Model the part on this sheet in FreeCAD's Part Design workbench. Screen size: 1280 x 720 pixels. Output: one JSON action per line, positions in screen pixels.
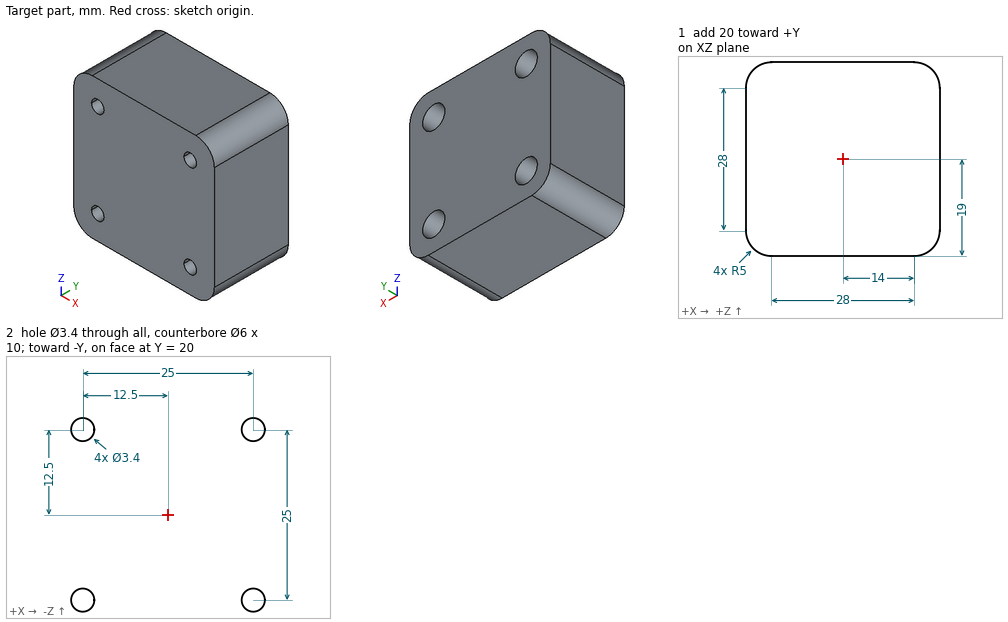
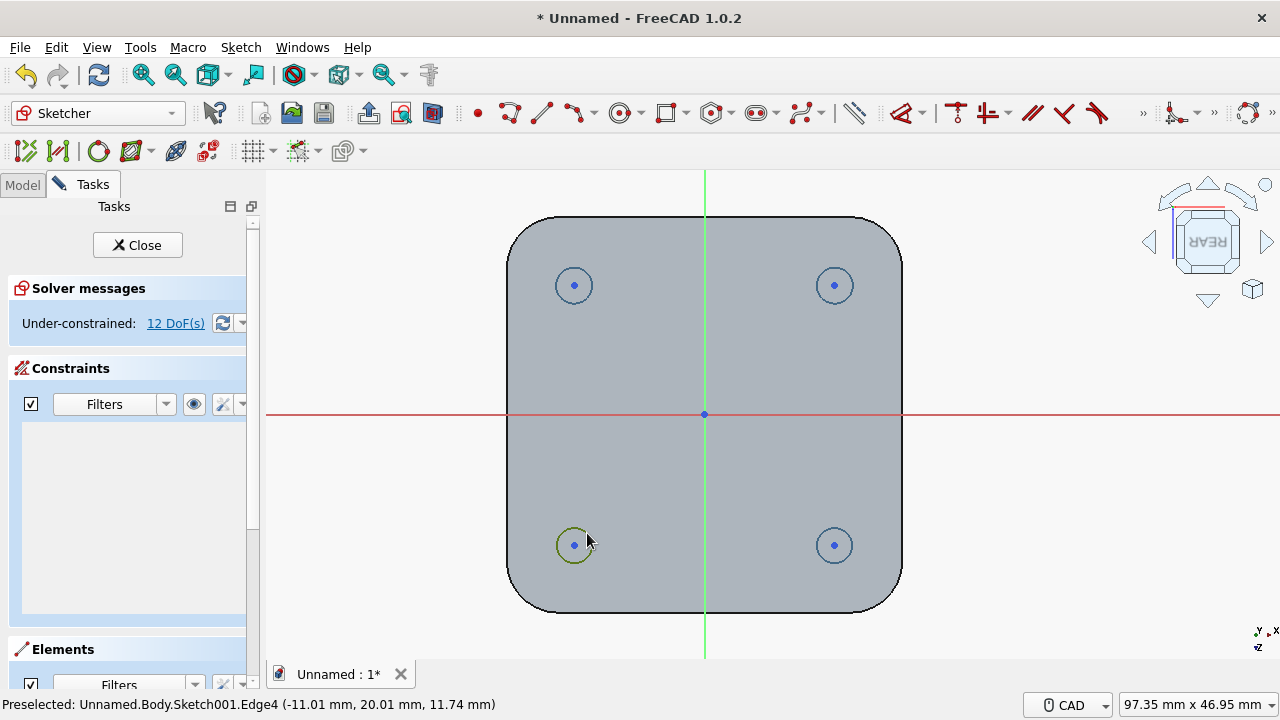
{"action": "key", "text": "e"}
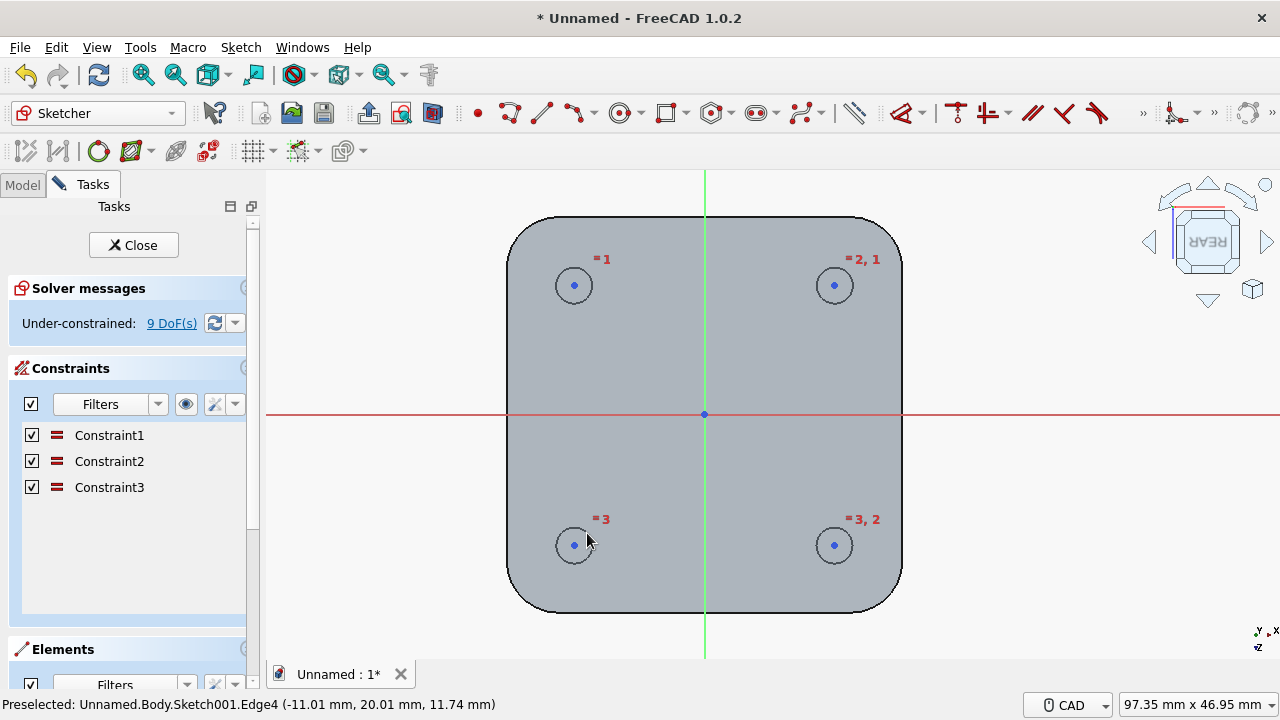
{"action": "left_click", "coordinate": [574, 286]}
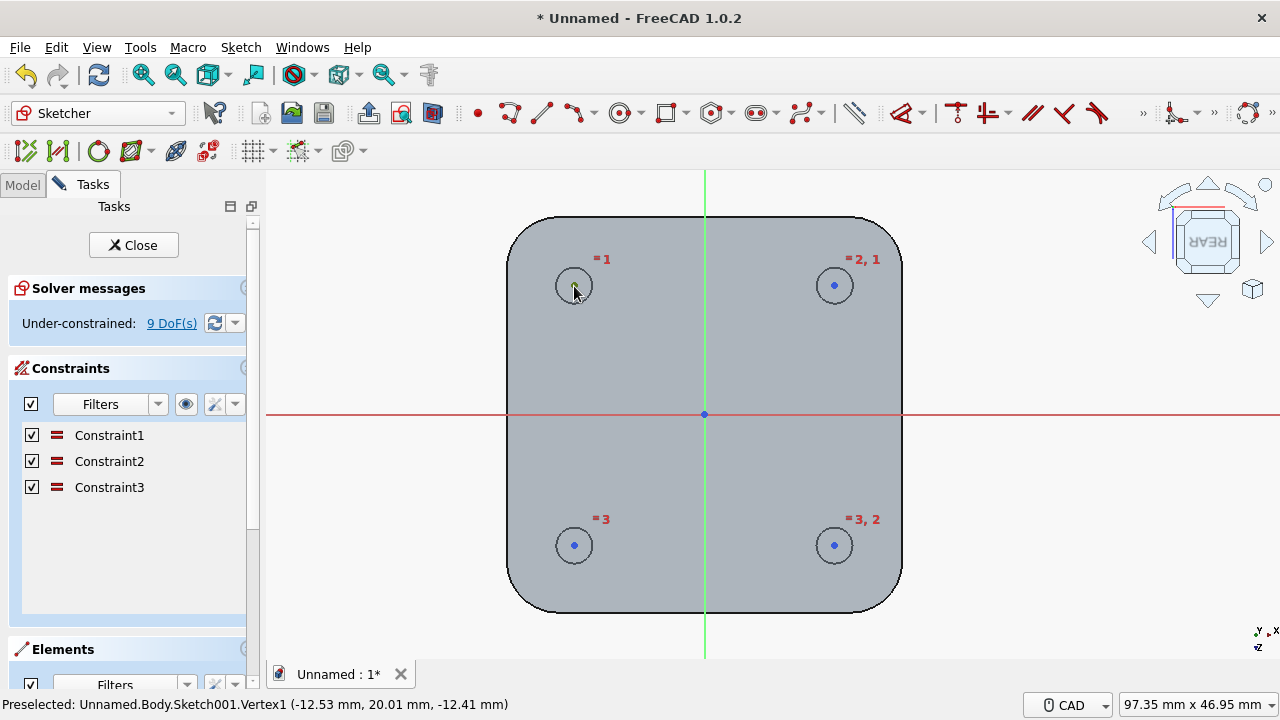
{"action": "left_click", "coordinate": [835, 286]}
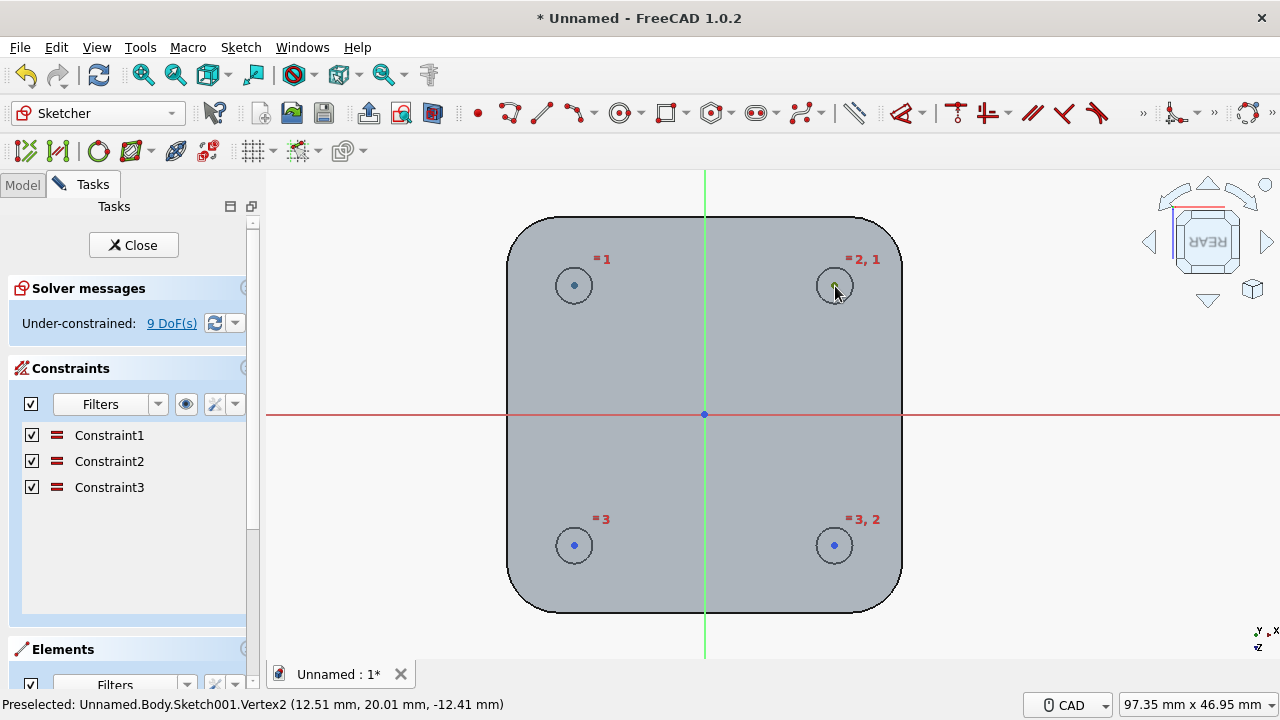
{"action": "left_click", "coordinate": [1010, 114]}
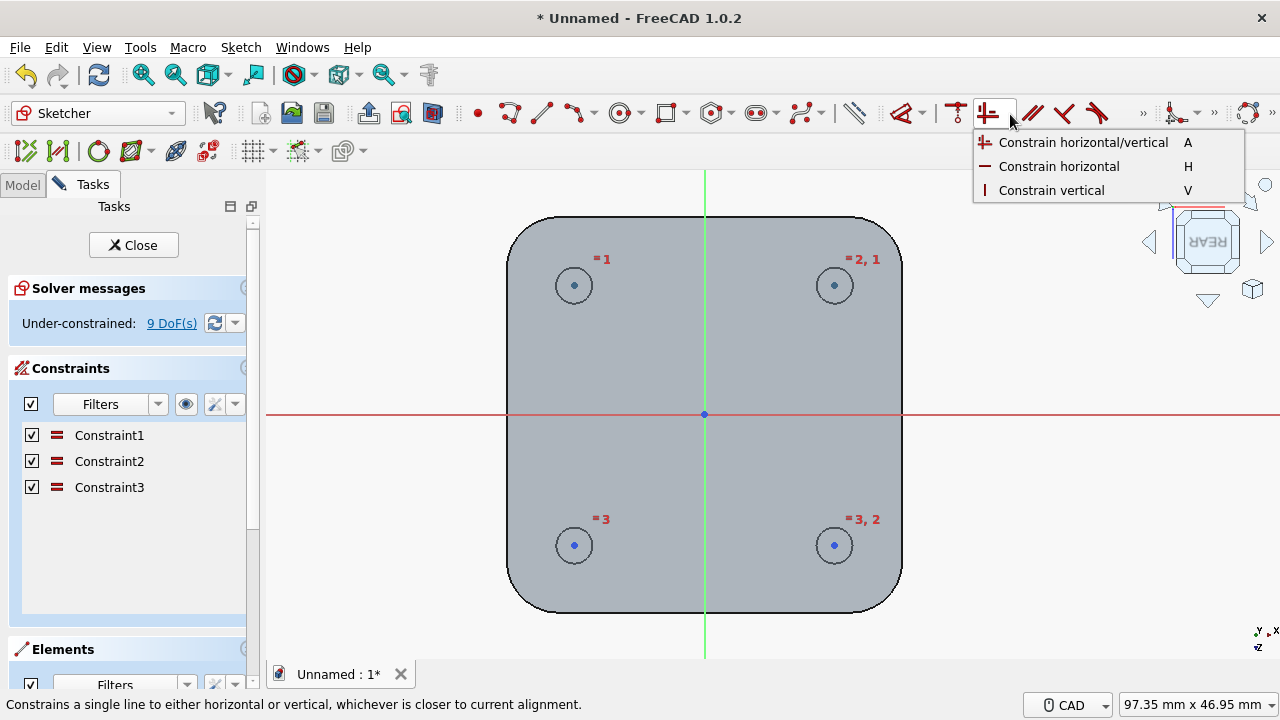
{"action": "left_click", "coordinate": [1109, 166]}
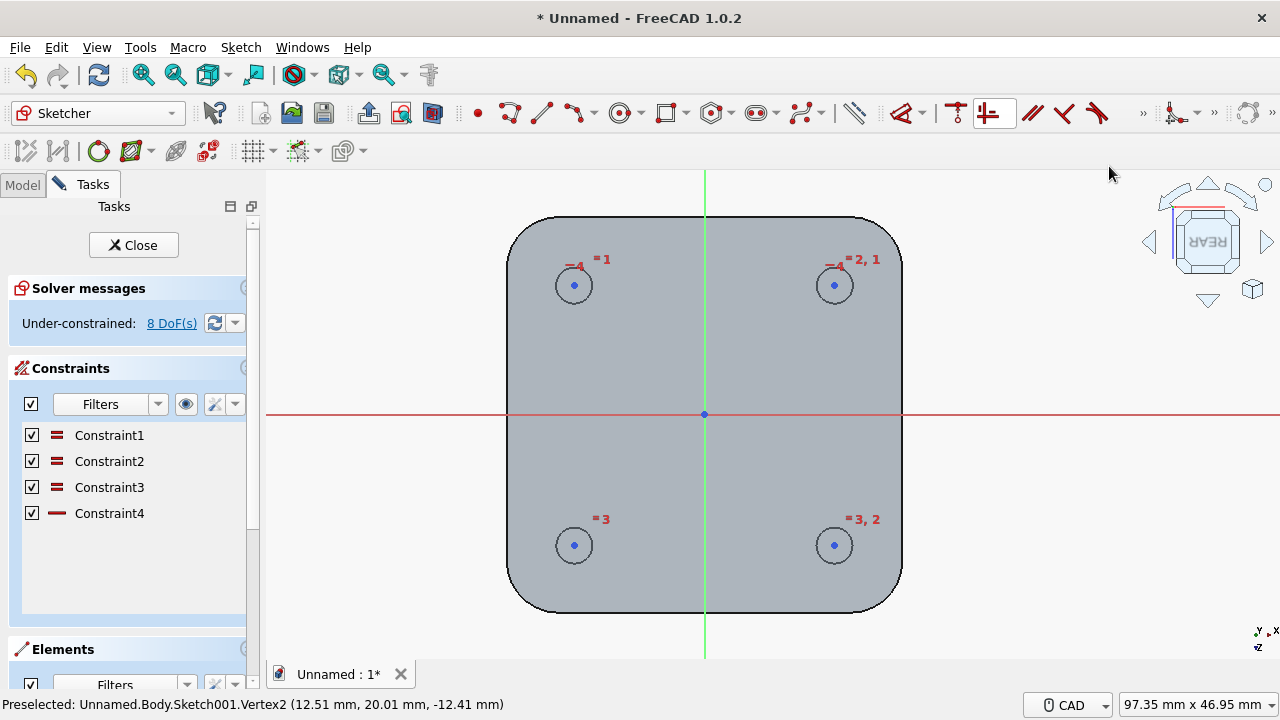
{"action": "left_click", "coordinate": [835, 286]}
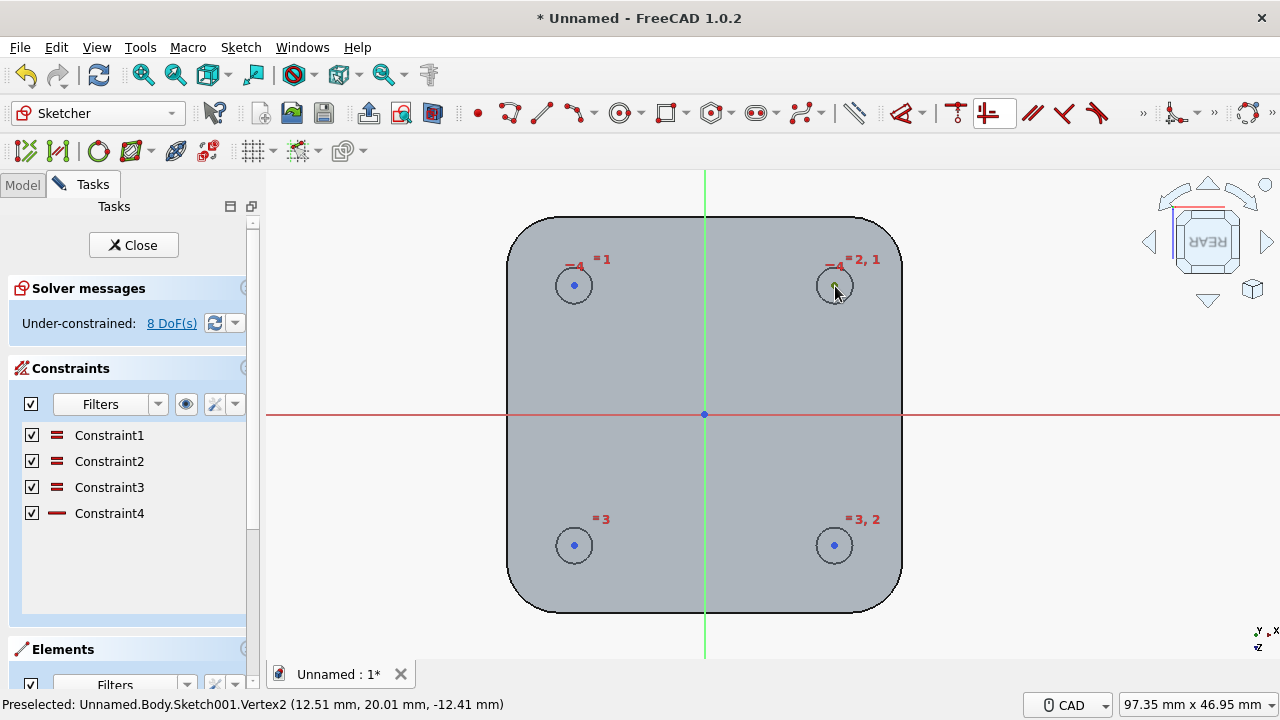
{"action": "left_click", "coordinate": [835, 546]}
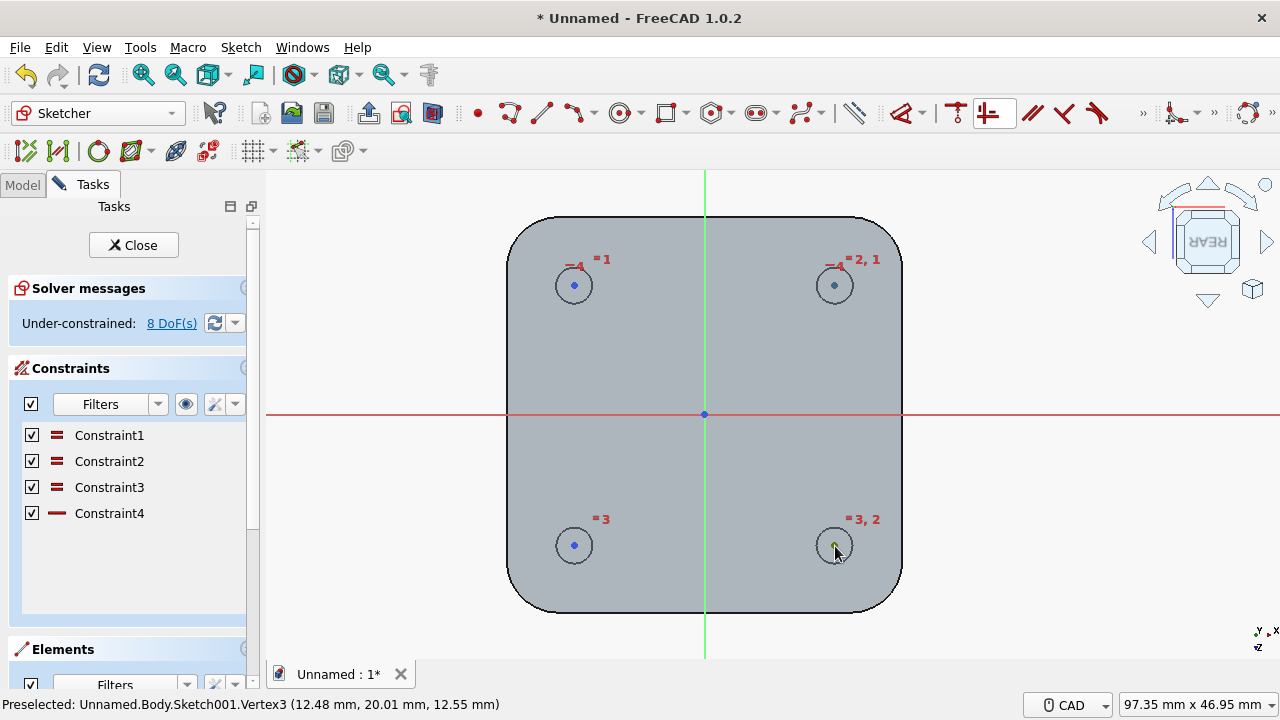
{"action": "key", "text": "v"}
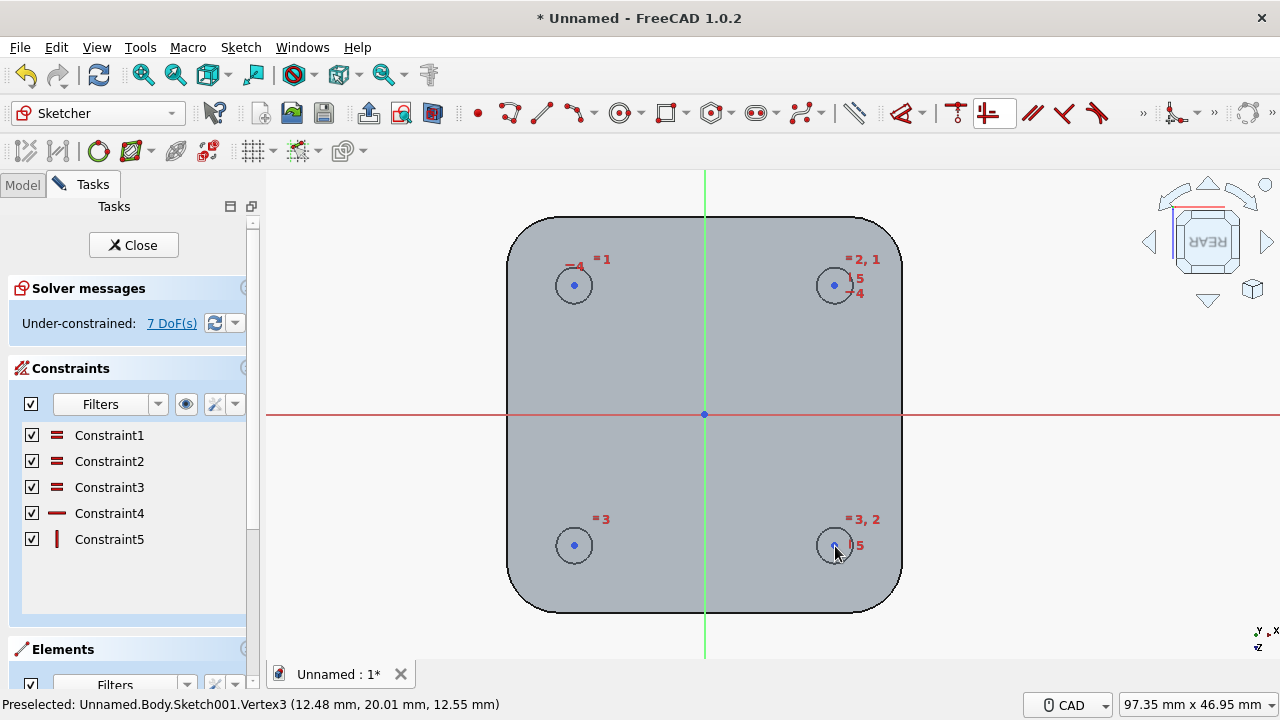
{"action": "left_click", "coordinate": [574, 286]}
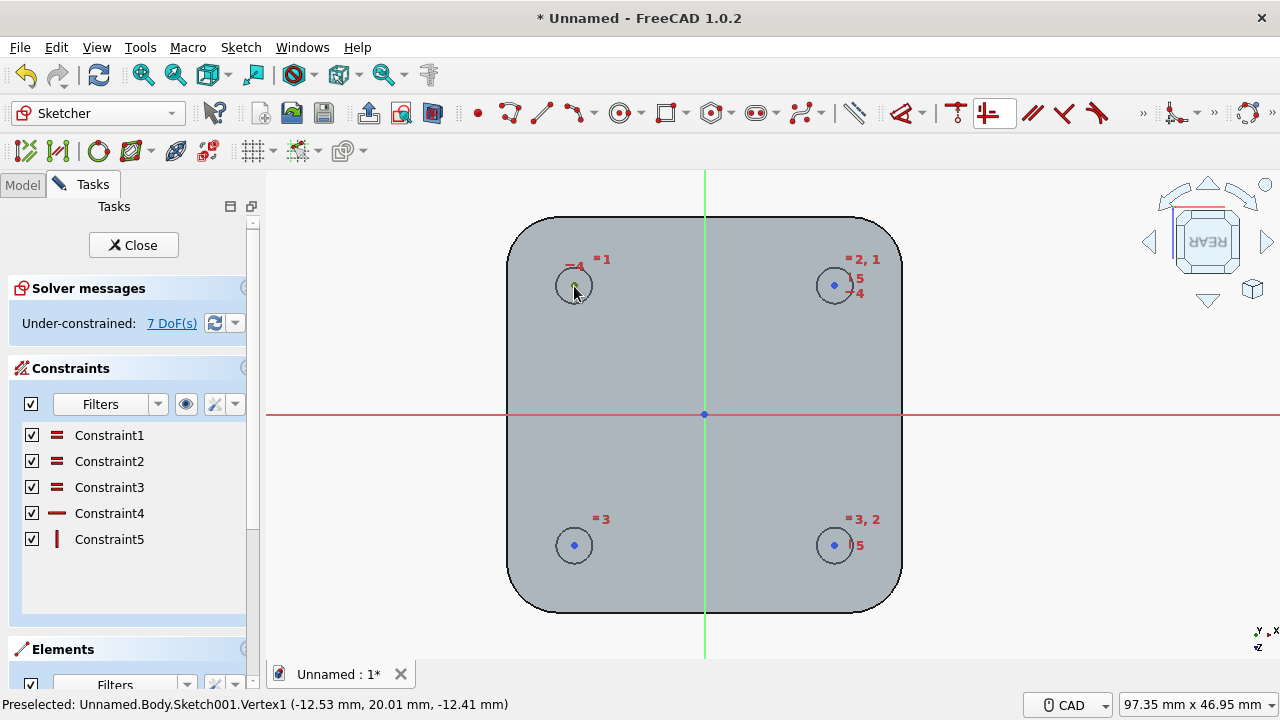
{"action": "left_click", "coordinate": [574, 546]}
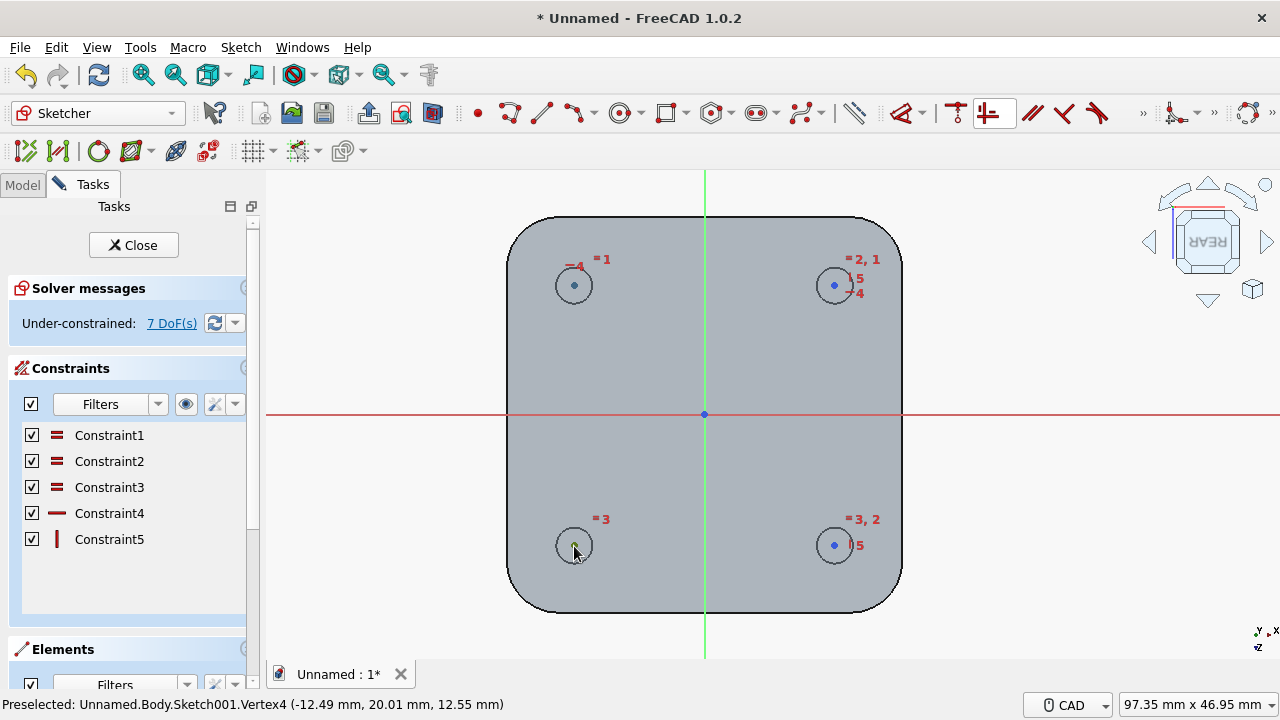
{"action": "left_click", "coordinate": [1010, 114]}